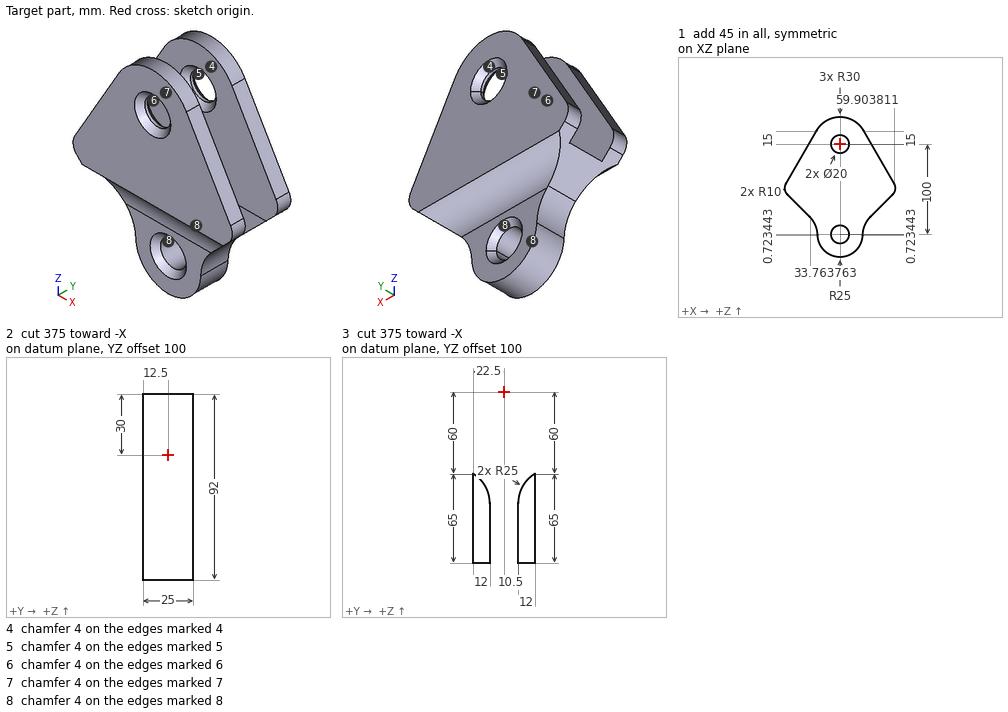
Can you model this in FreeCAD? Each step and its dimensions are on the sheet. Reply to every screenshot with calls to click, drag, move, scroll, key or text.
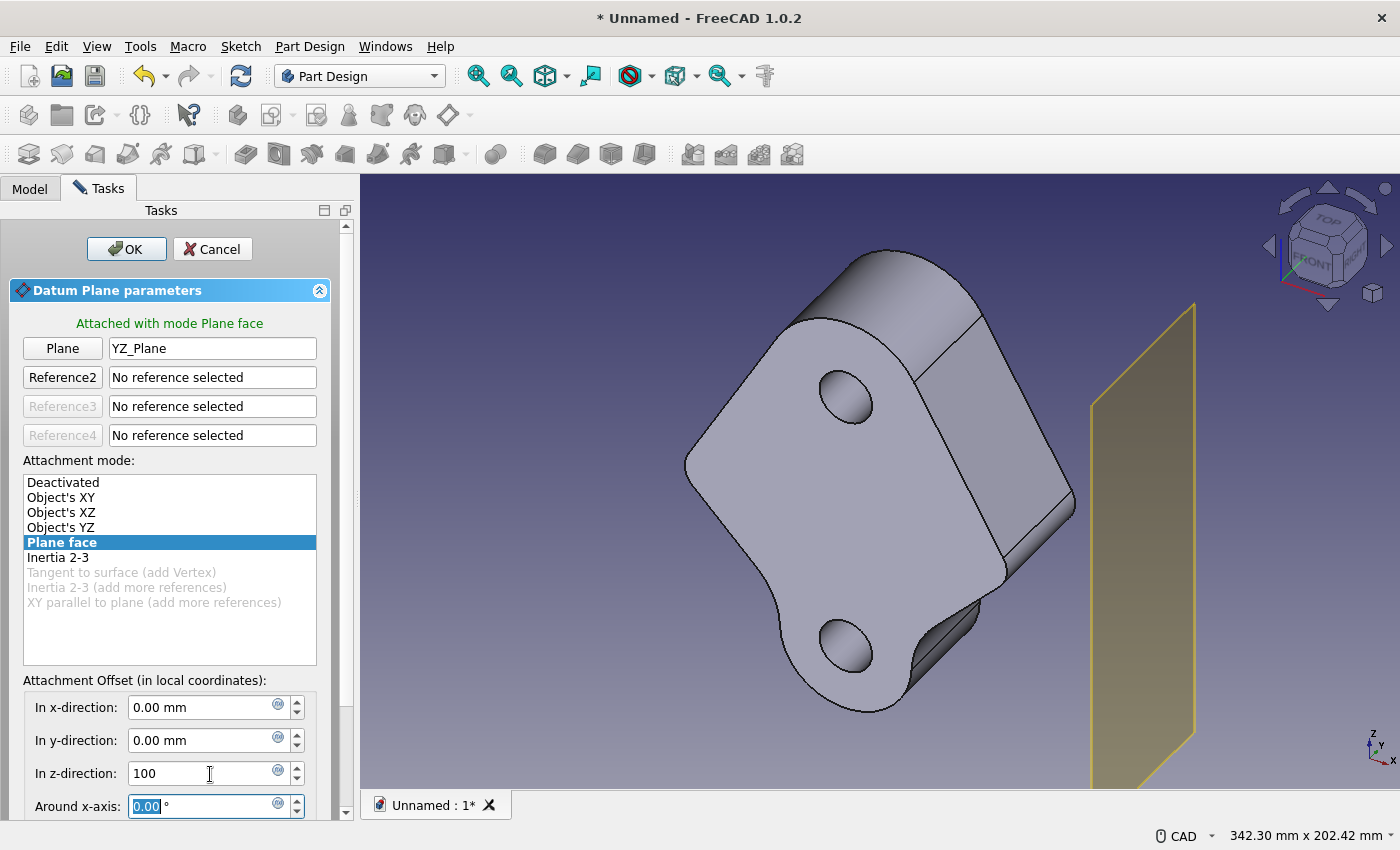
click(127, 249)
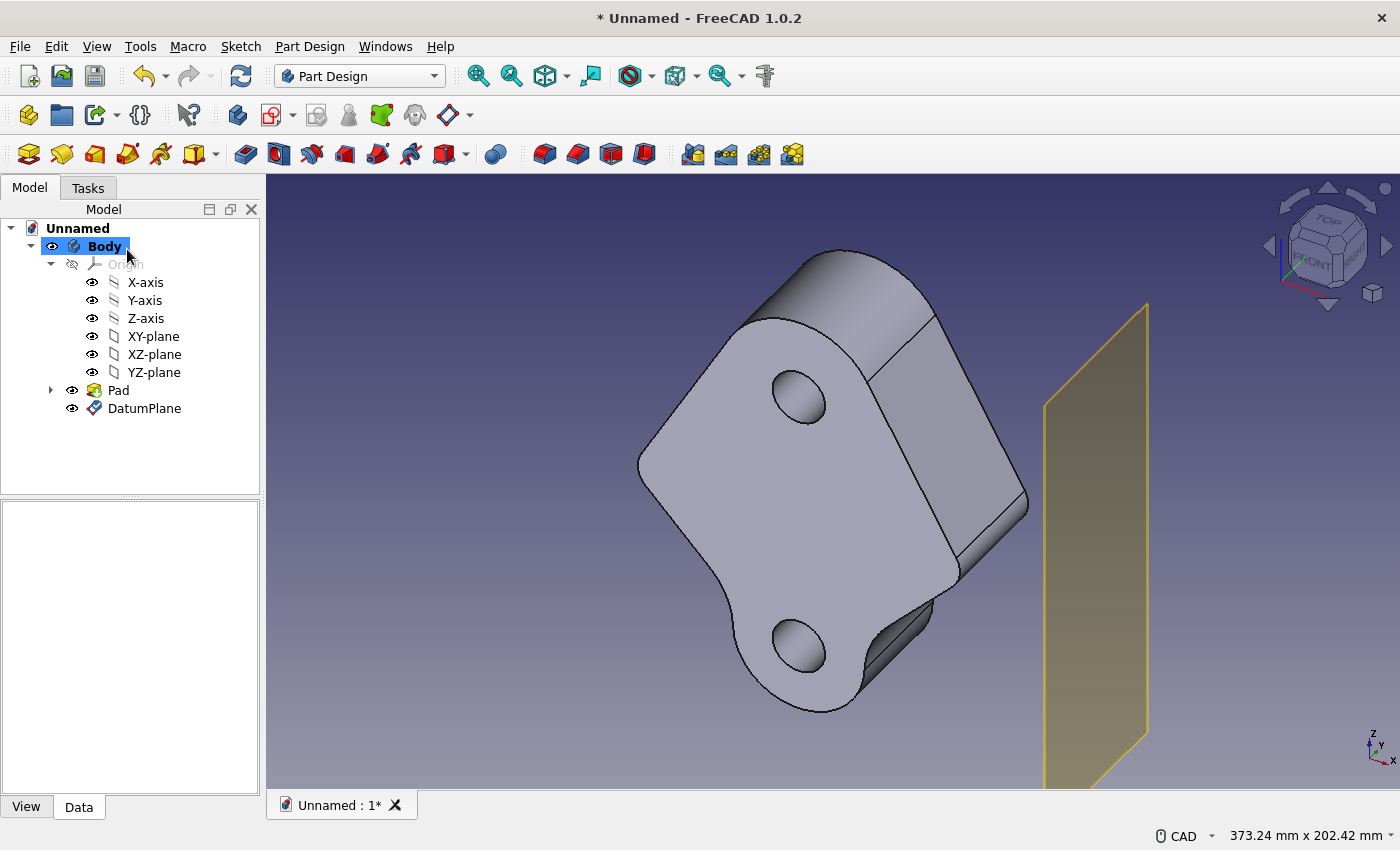
click(117, 408)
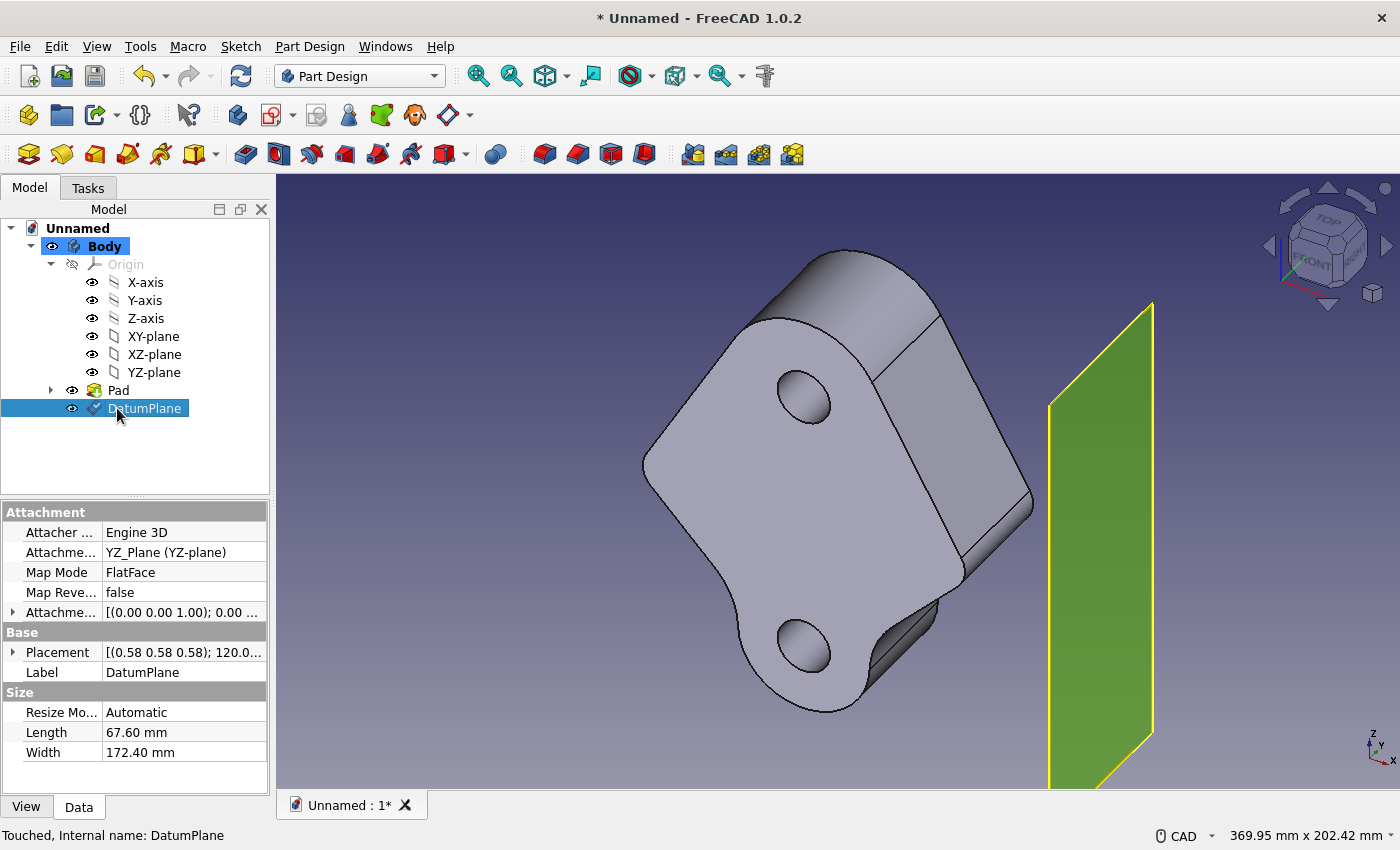
click(270, 116)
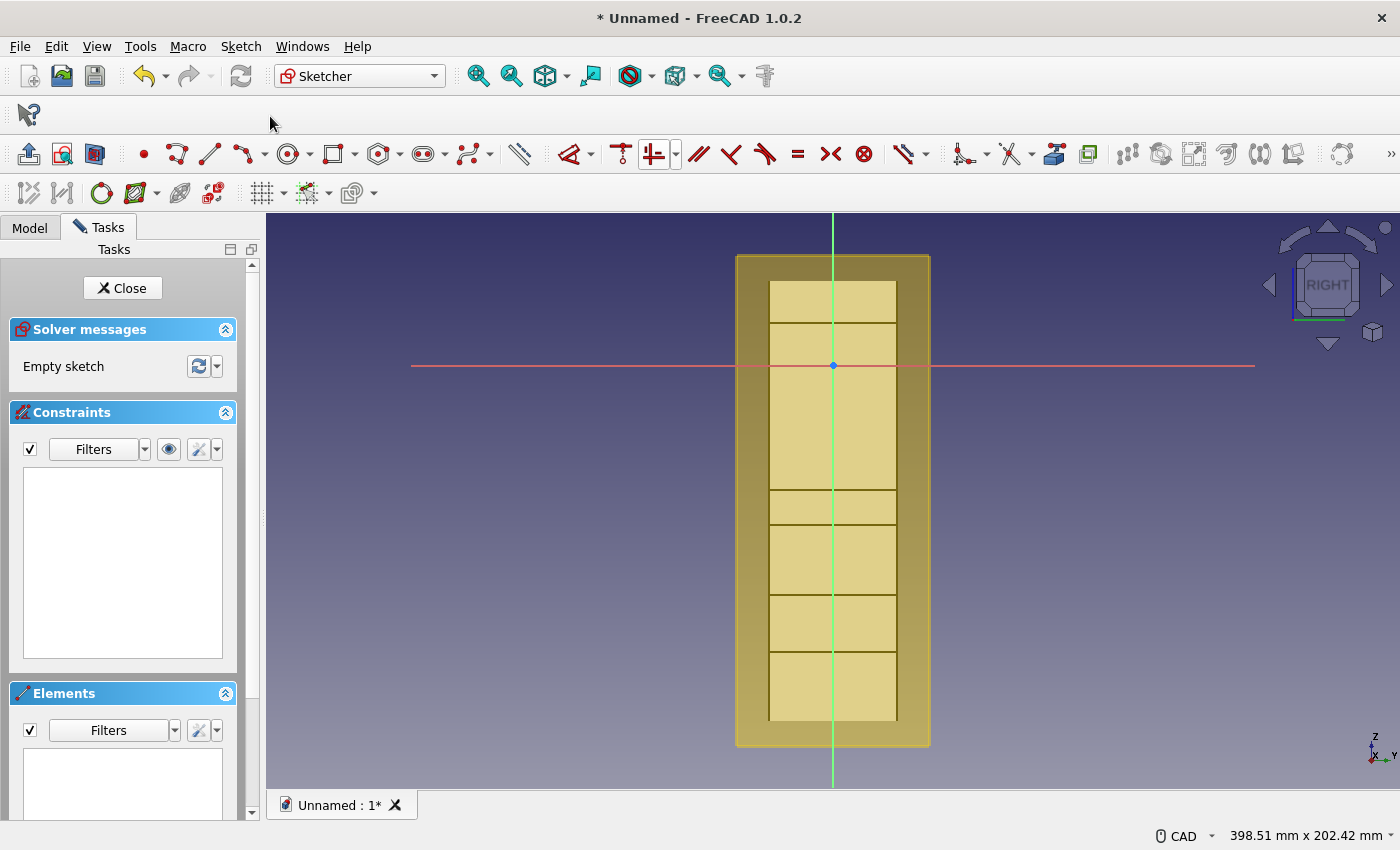
scroll(972, 241, up, 2)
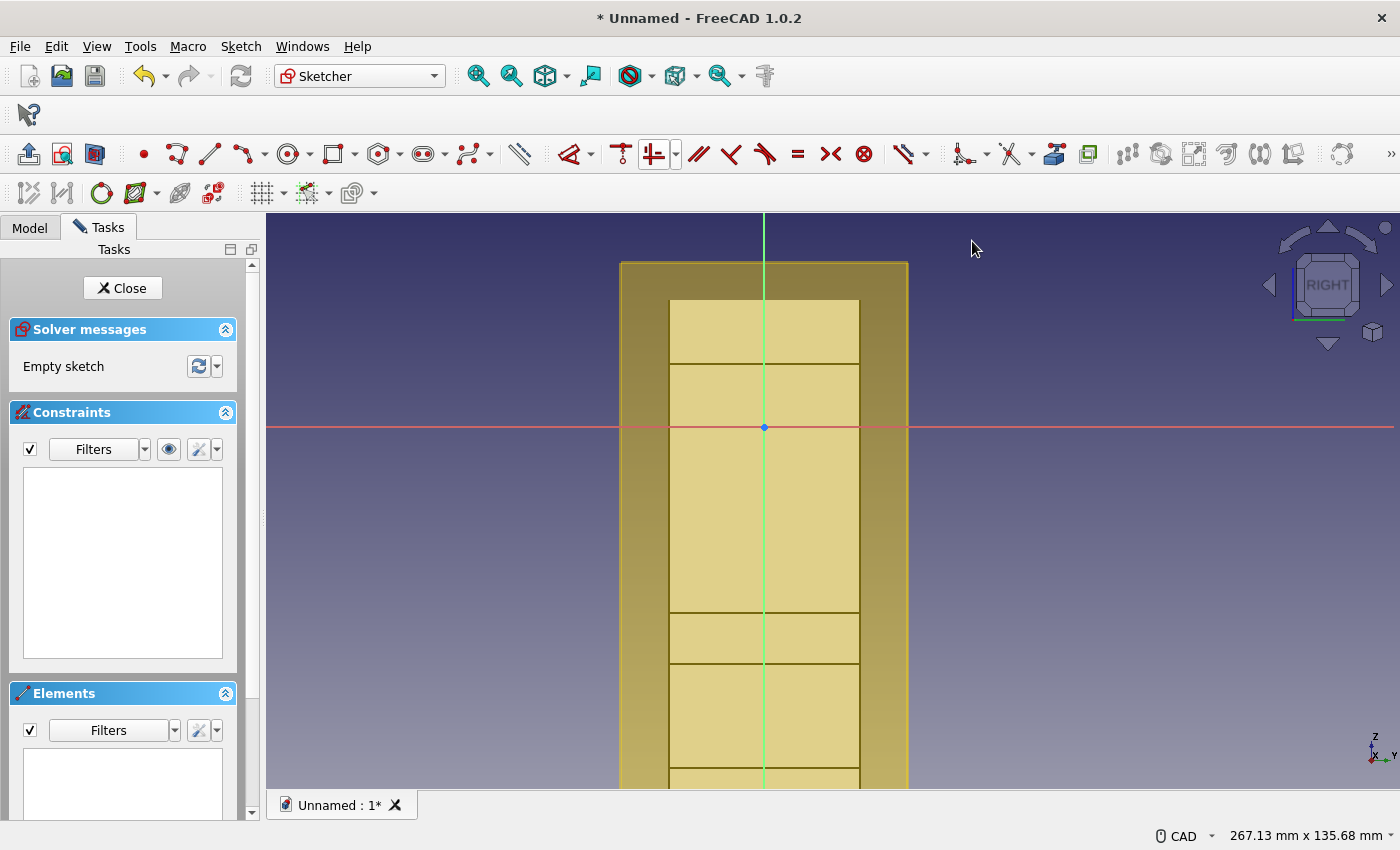
click(332, 154)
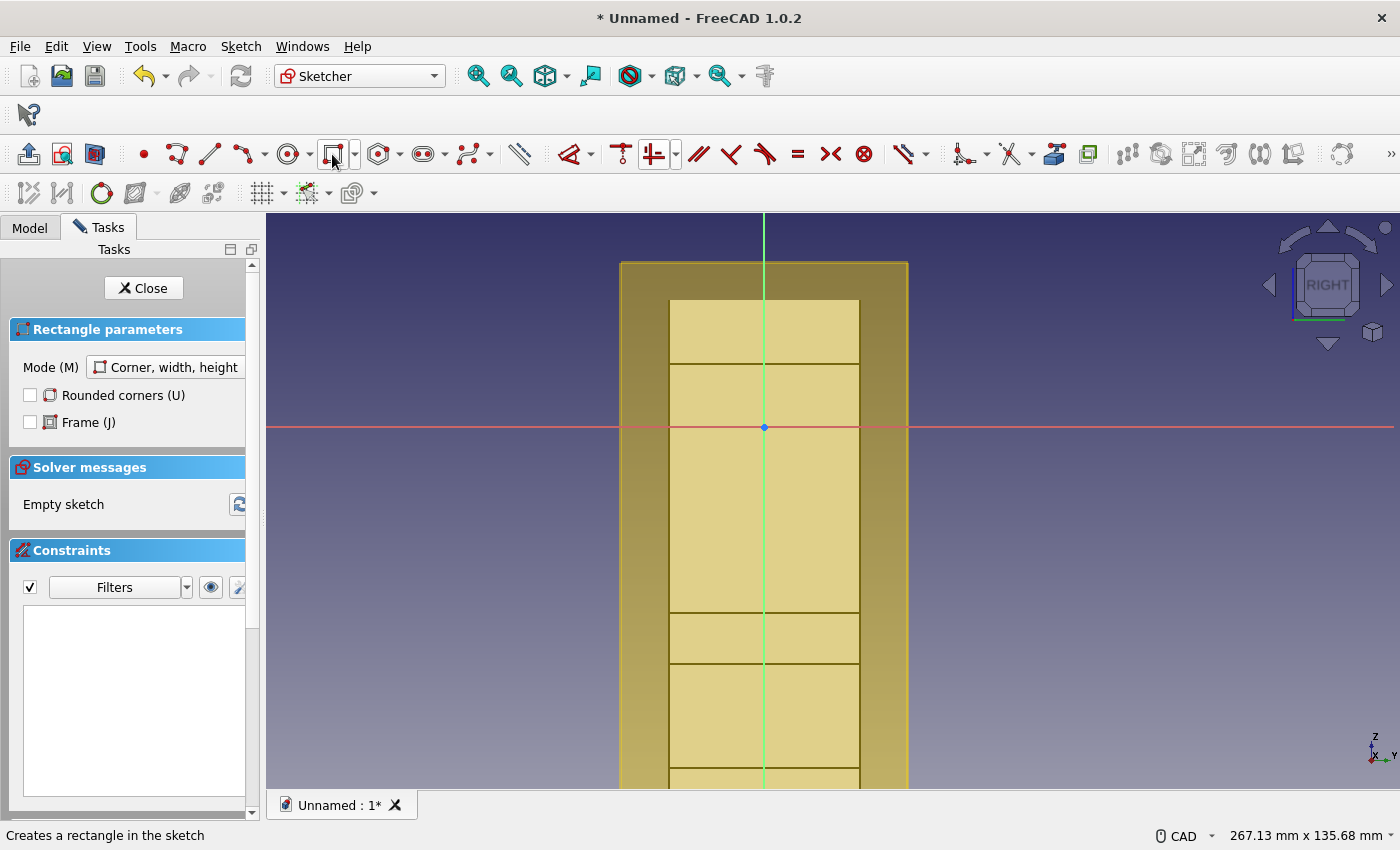
click(711, 300)
move(817, 690)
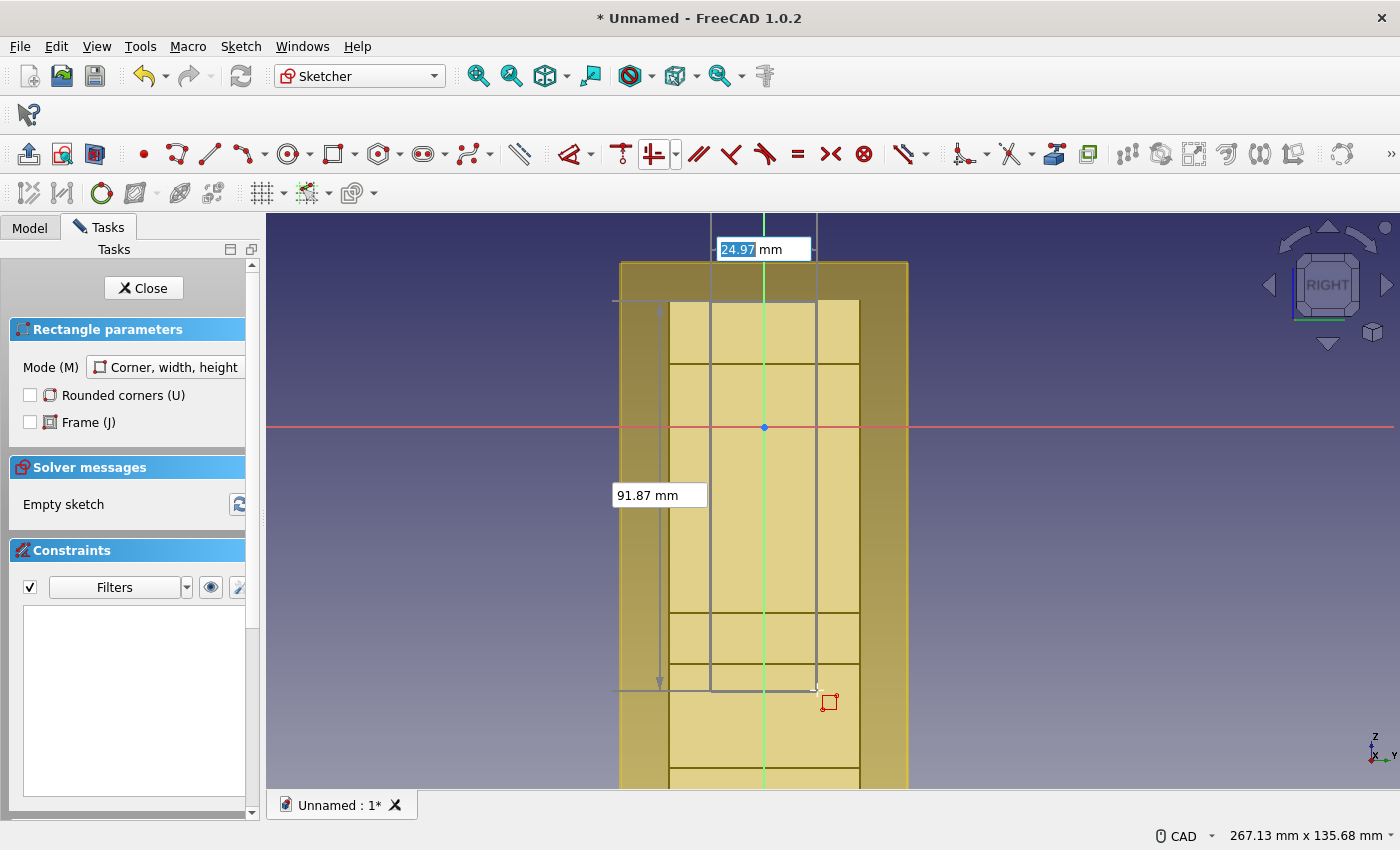
text(25)
key(Tab)
text(92)
key(Return)
key(Escape)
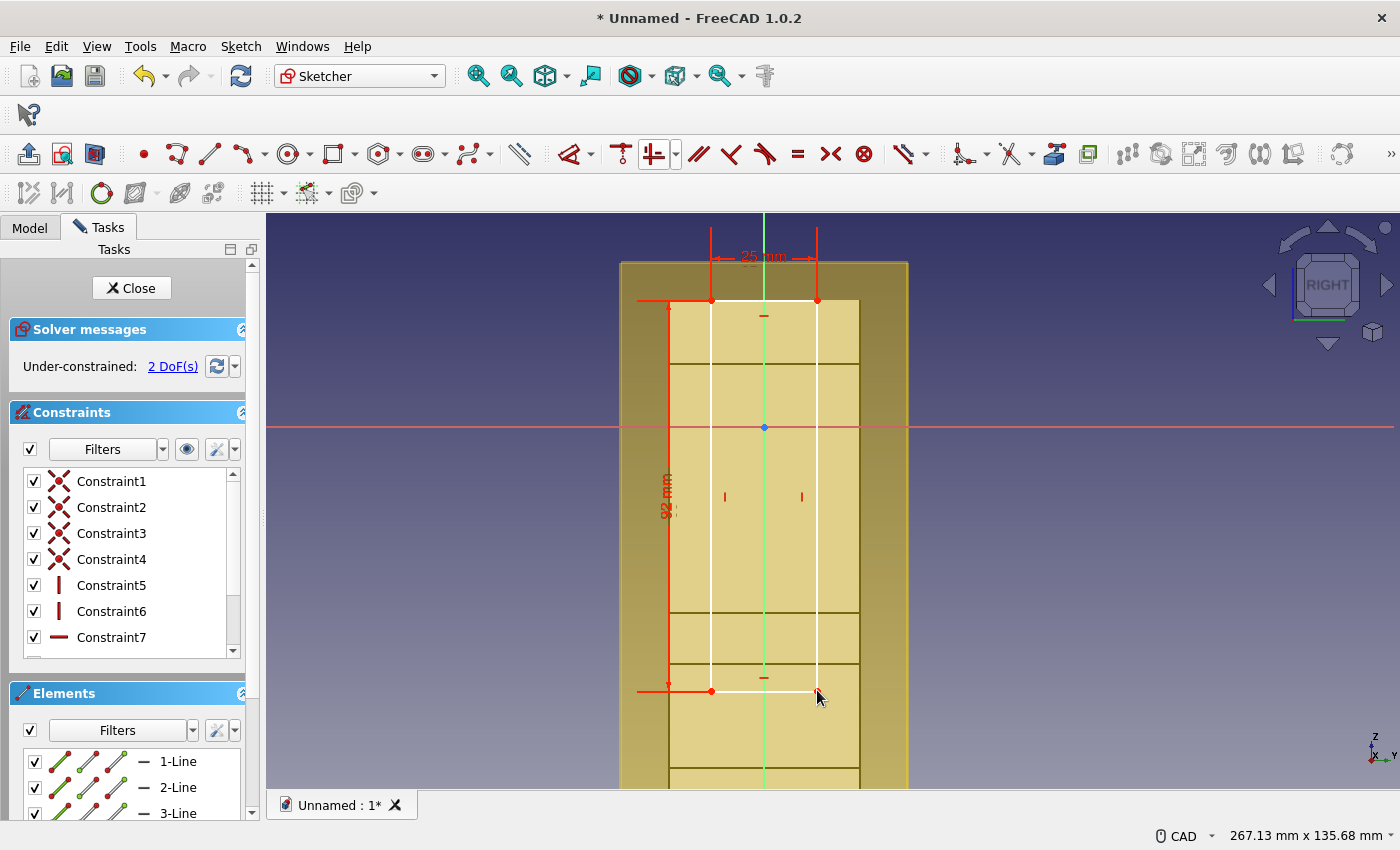
click(568, 154)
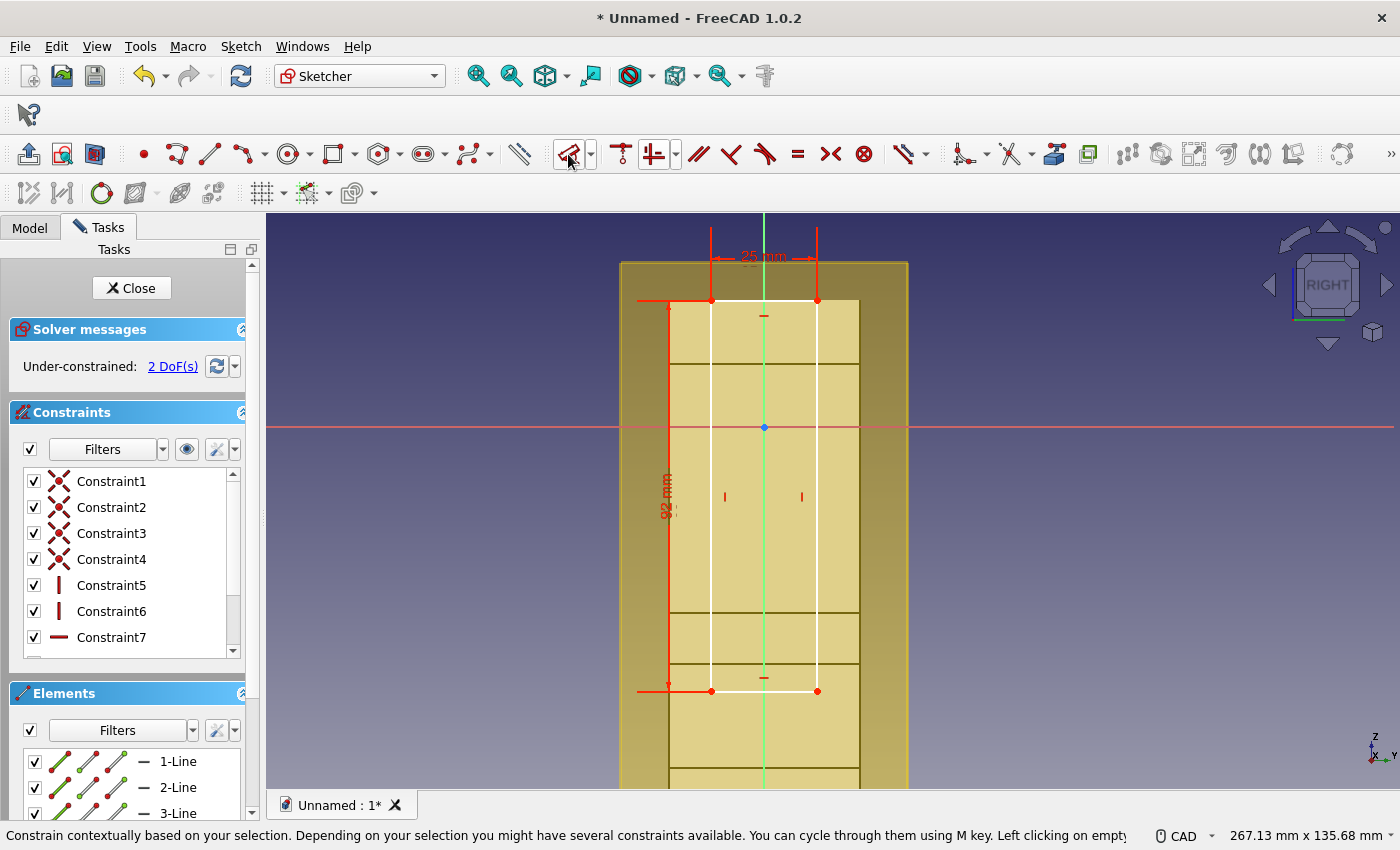
click(711, 301)
click(677, 364)